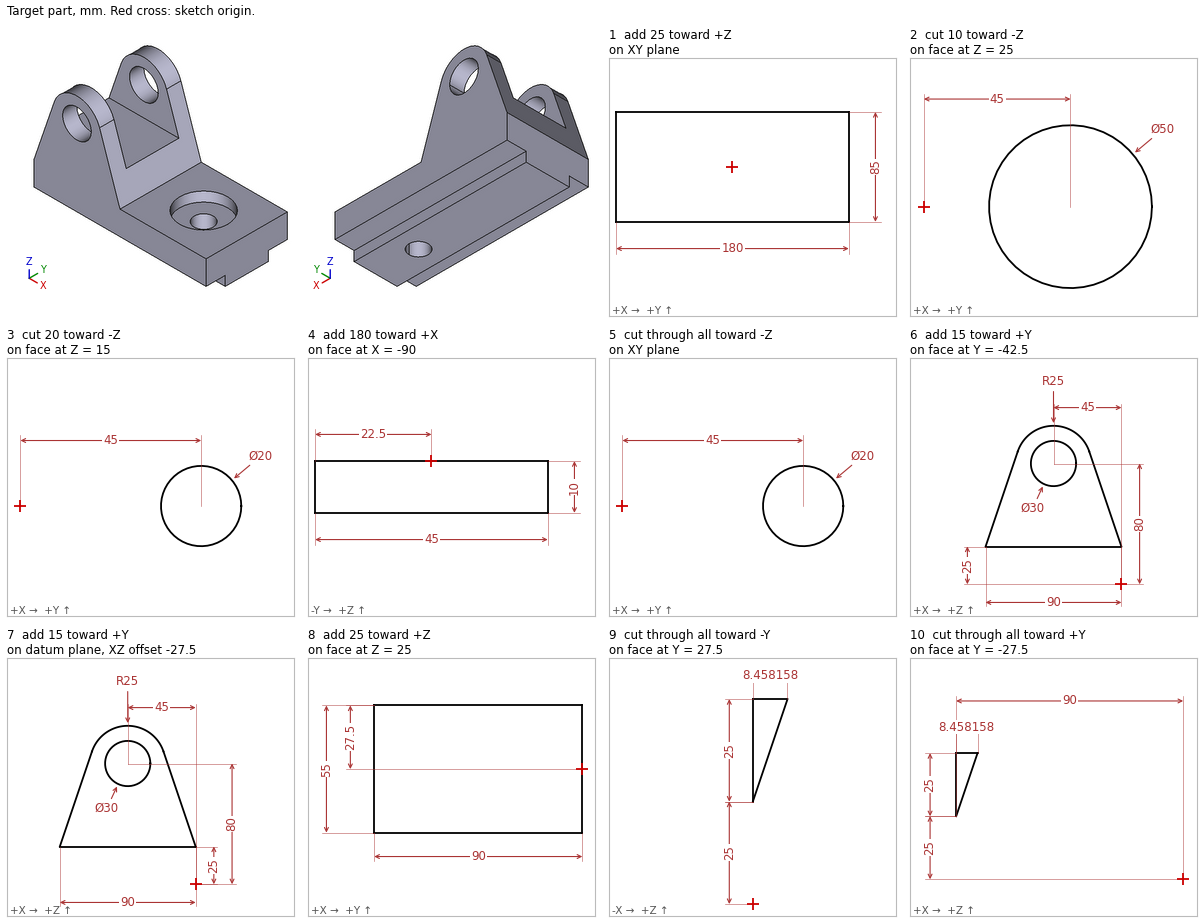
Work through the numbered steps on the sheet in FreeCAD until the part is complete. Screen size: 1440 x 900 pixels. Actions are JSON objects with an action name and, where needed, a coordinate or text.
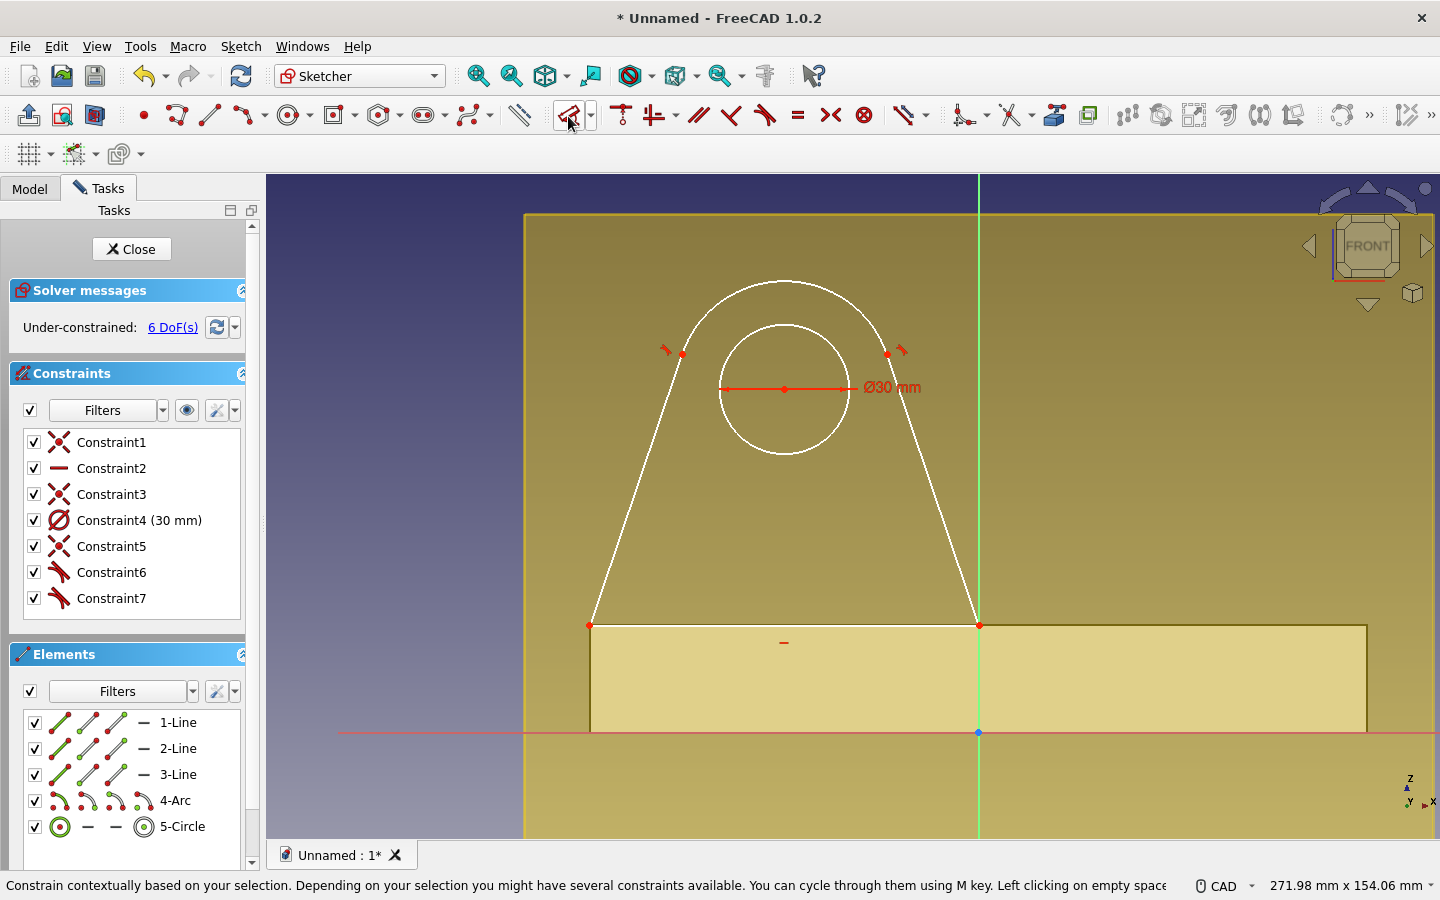
{"action": "left_click", "coordinate": [836, 294]}
{"action": "left_click", "coordinate": [851, 266]}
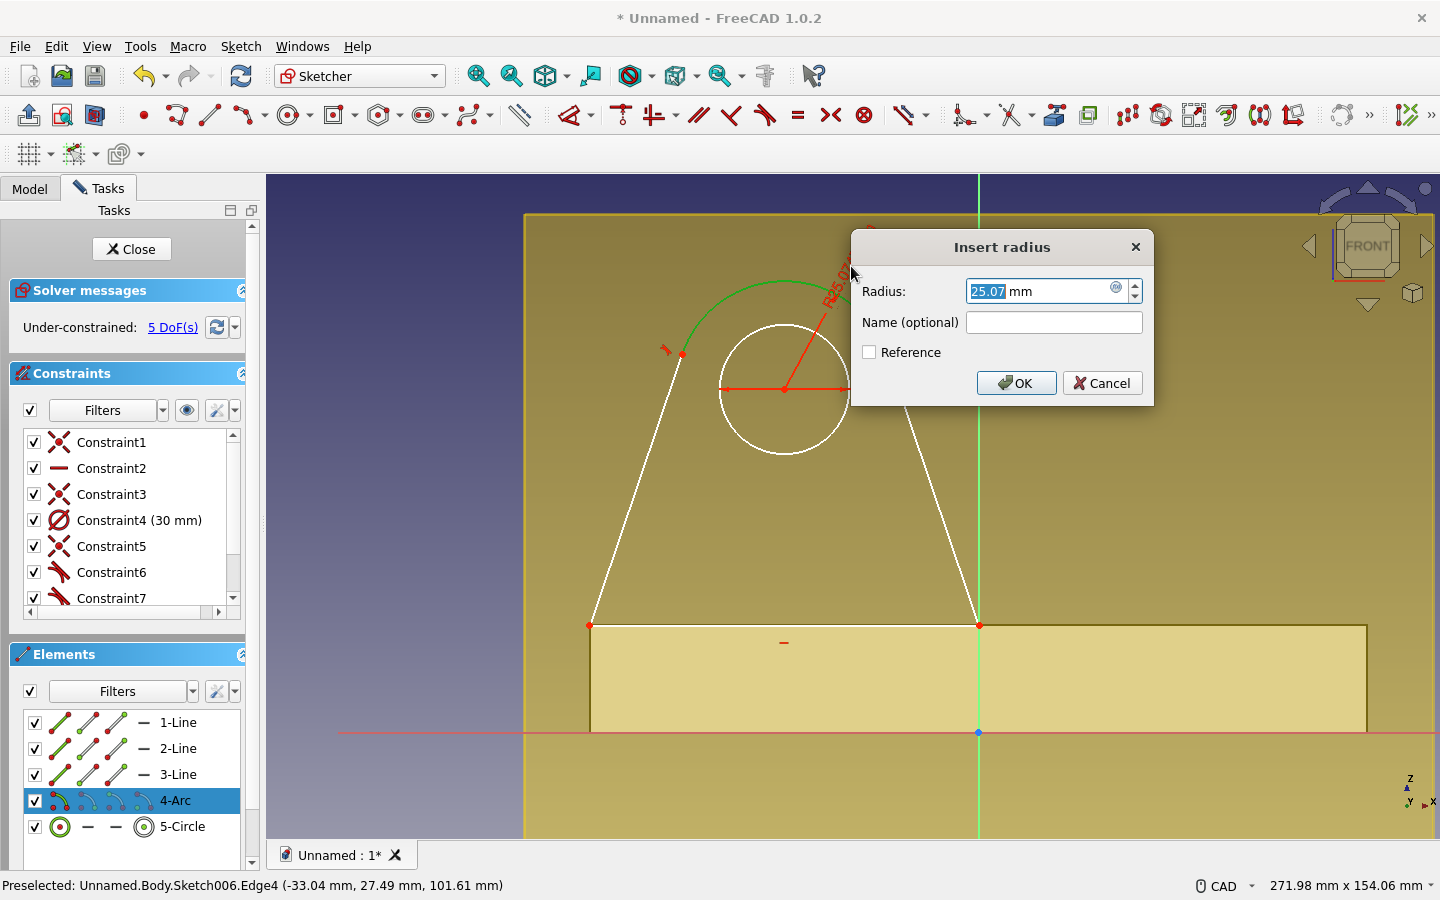
{"action": "type", "text": "25"}
{"action": "key", "text": "Return"}
{"action": "key", "text": "Escape"}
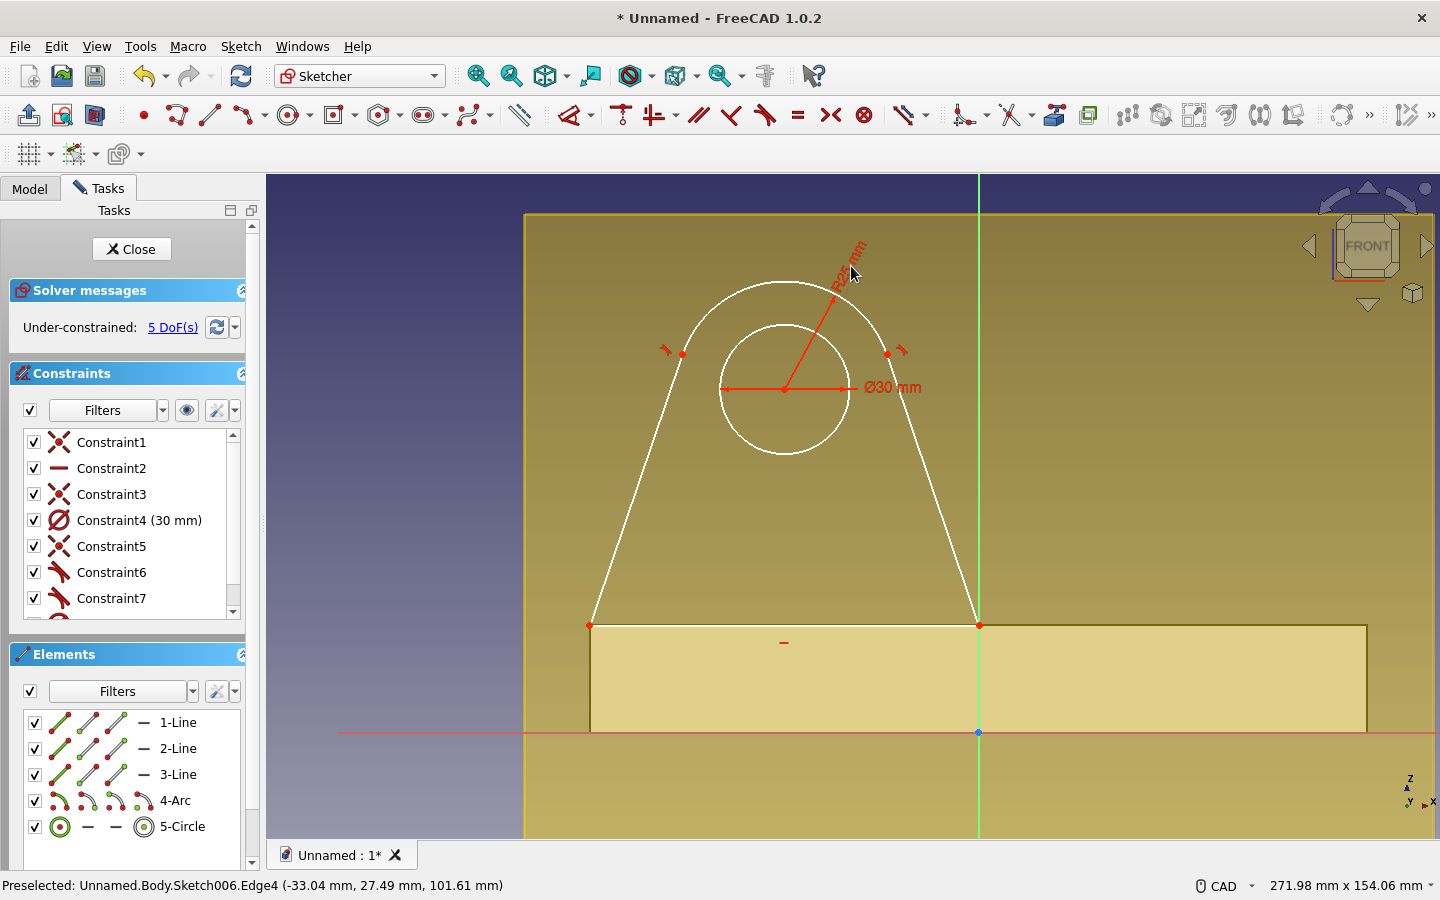
{"action": "left_click", "coordinate": [979, 626]}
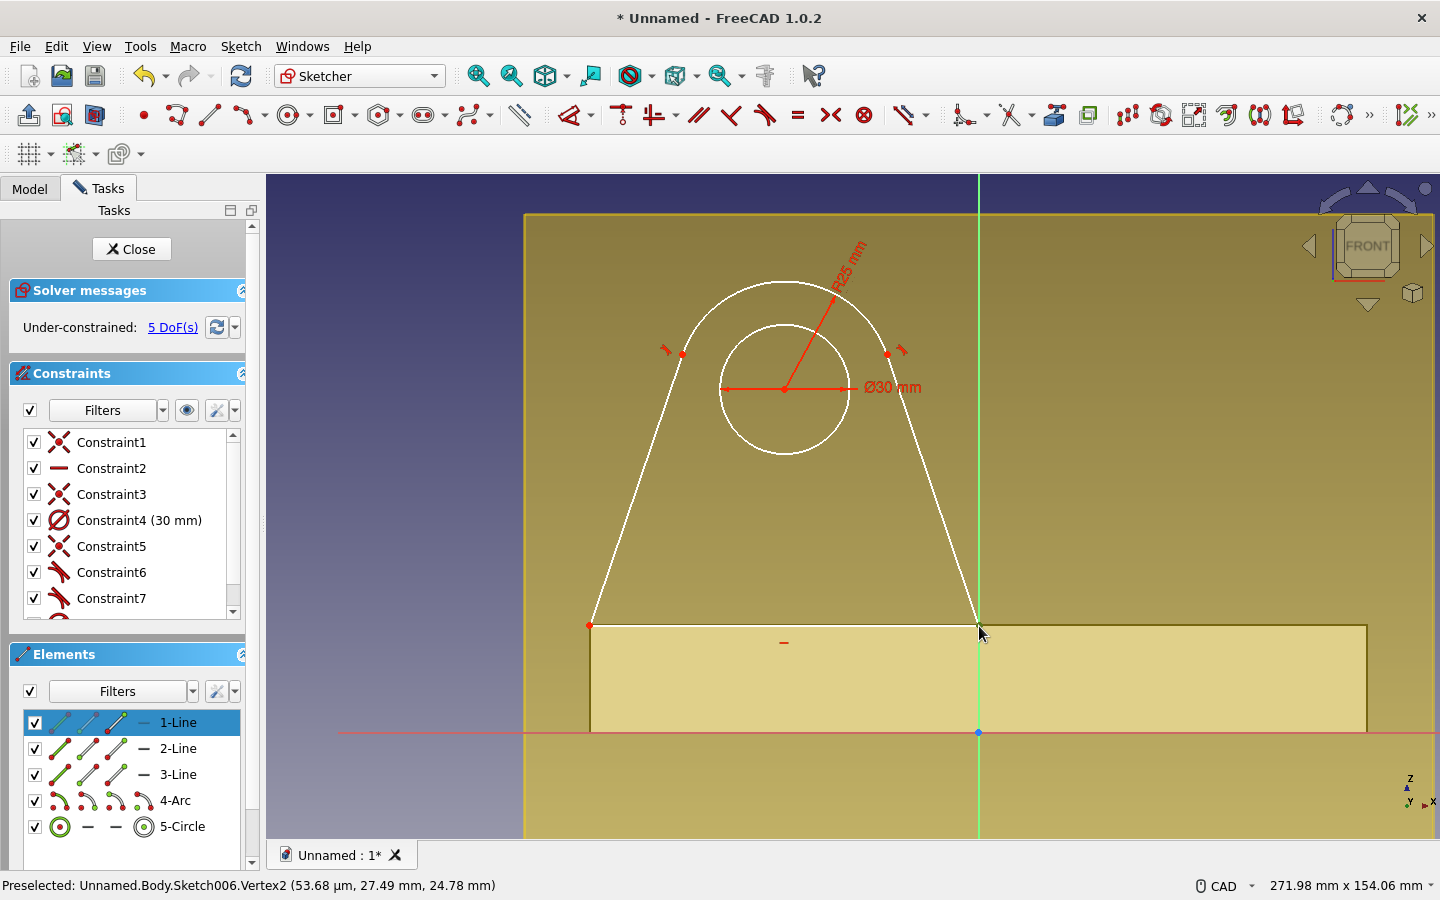
{"action": "left_click", "coordinate": [979, 768]}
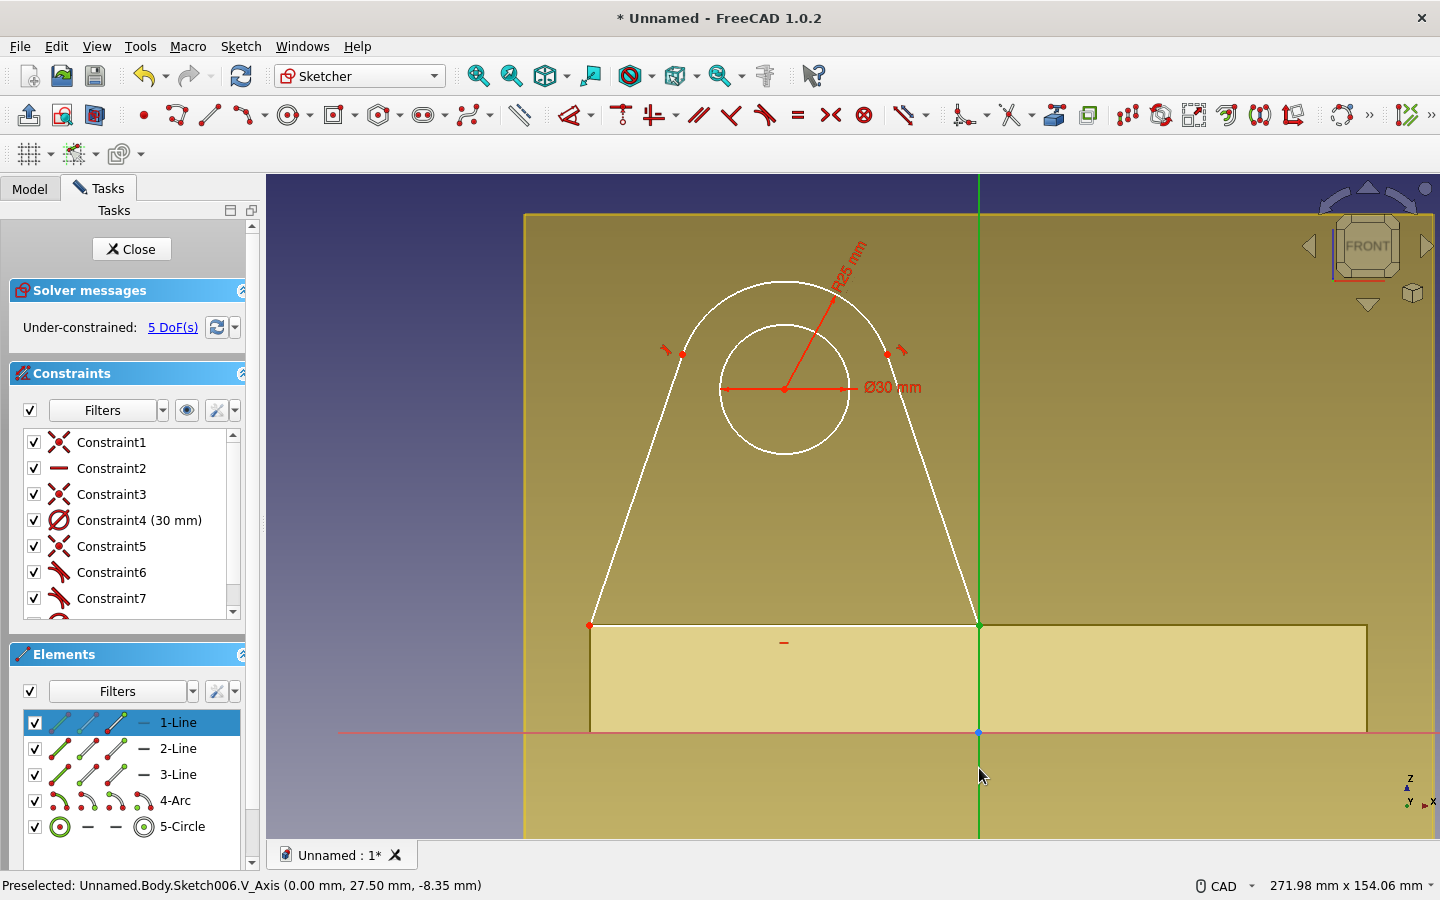
{"action": "left_click", "coordinate": [621, 116]}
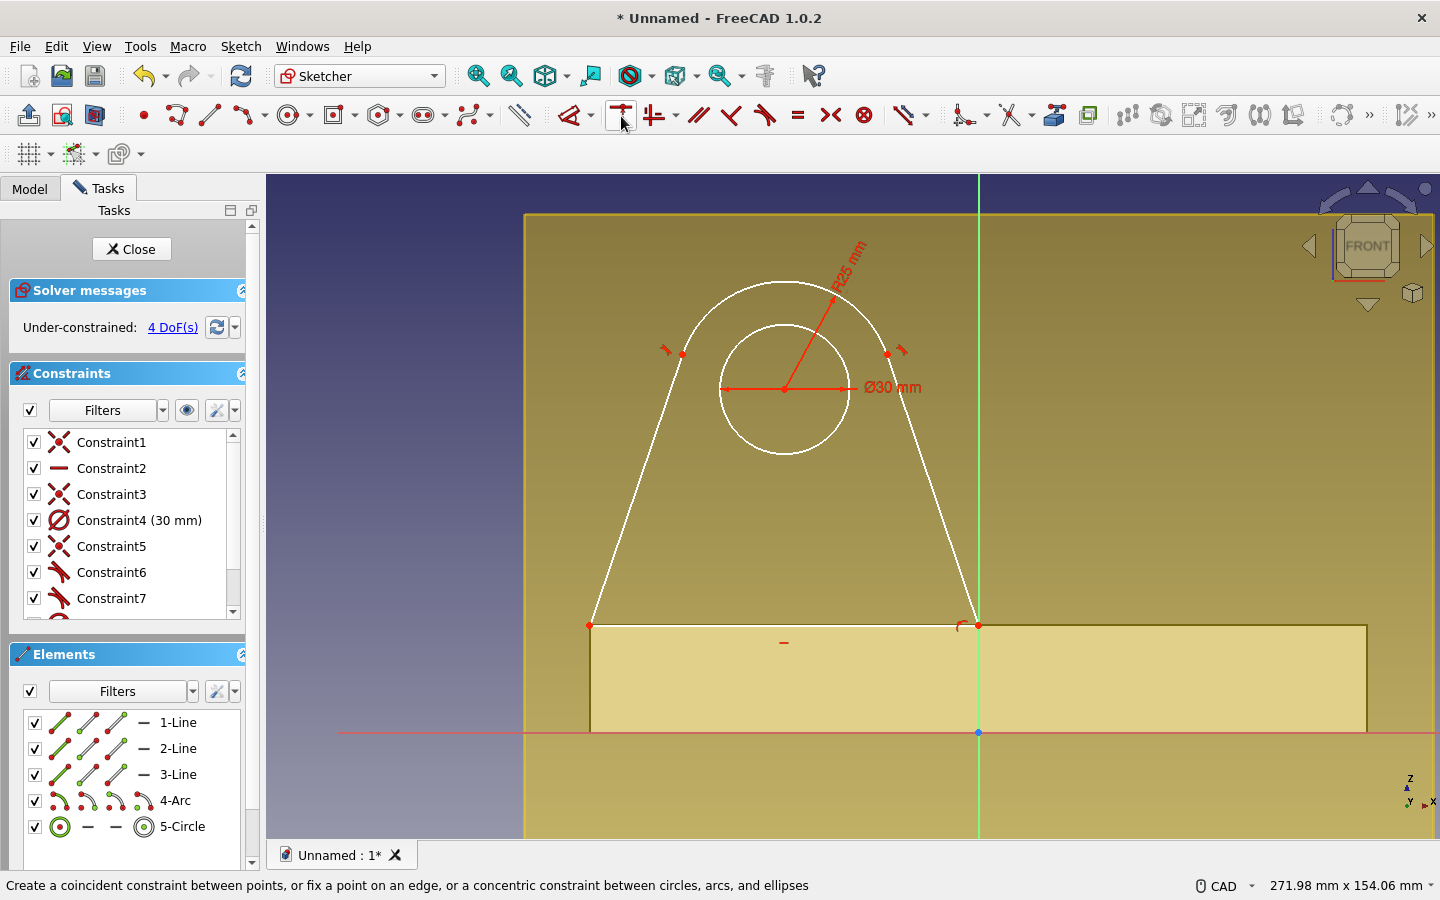
{"action": "left_click", "coordinate": [568, 116]}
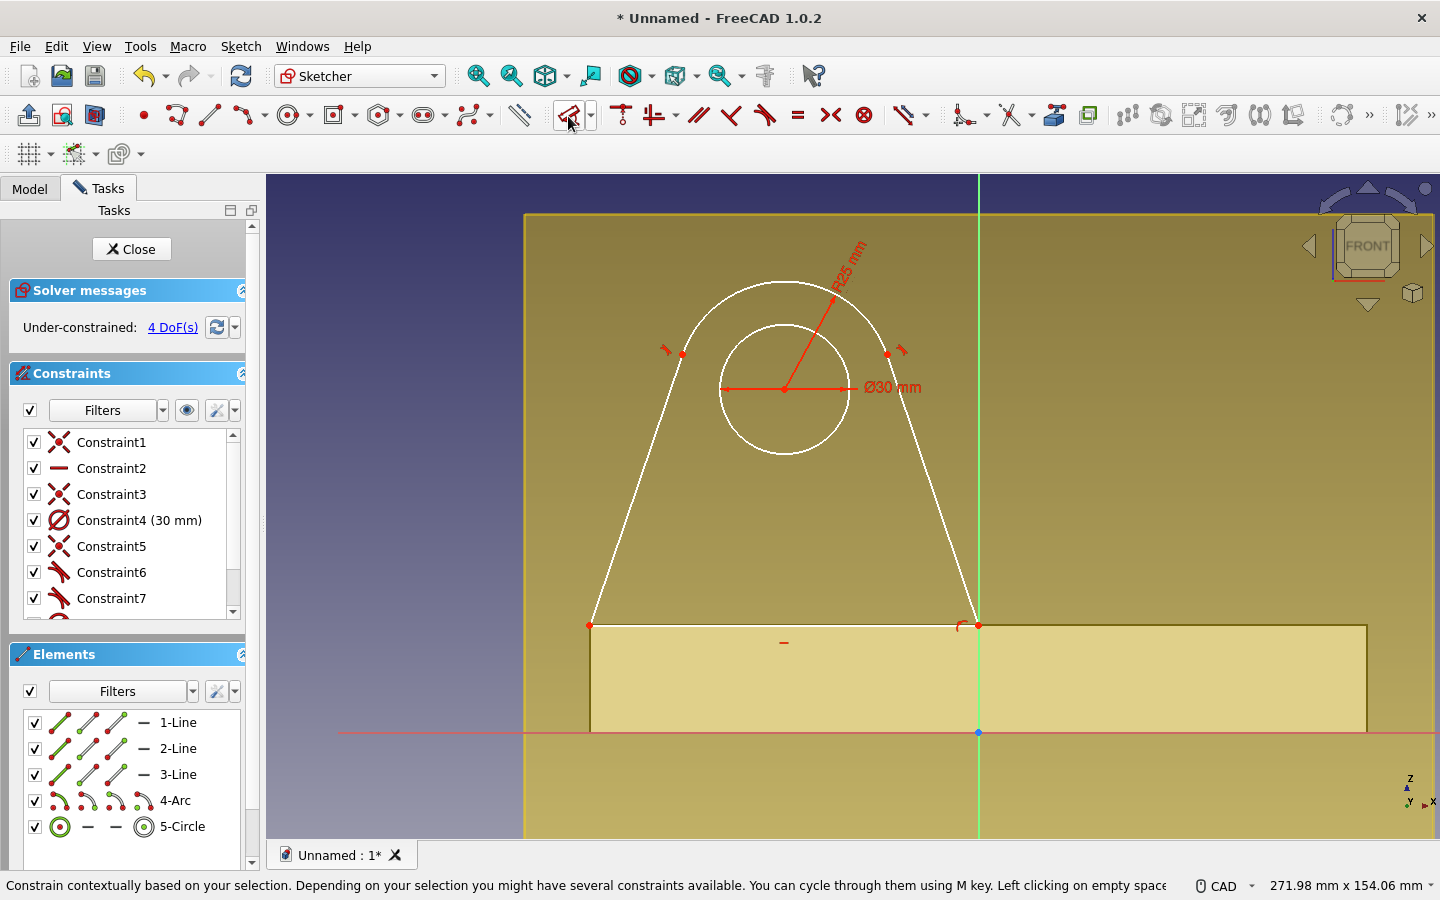
{"action": "left_click", "coordinate": [862, 626]}
{"action": "left_click", "coordinate": [784, 660]}